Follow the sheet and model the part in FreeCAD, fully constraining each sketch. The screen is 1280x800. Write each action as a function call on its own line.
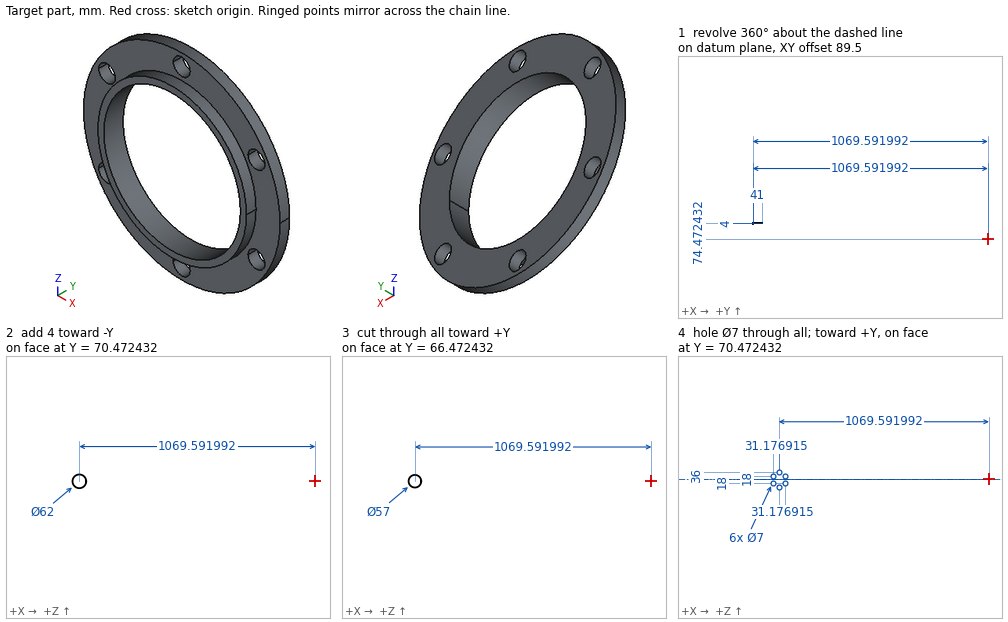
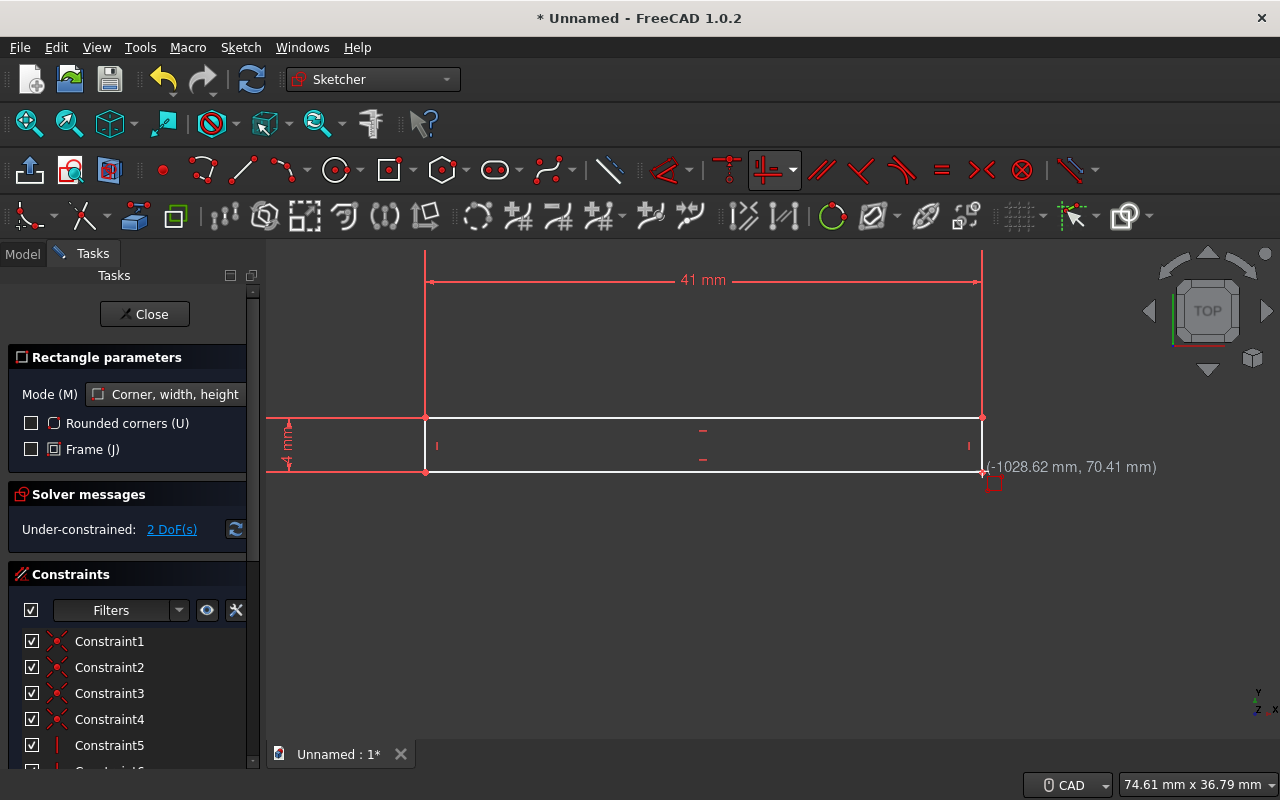
click(244, 170)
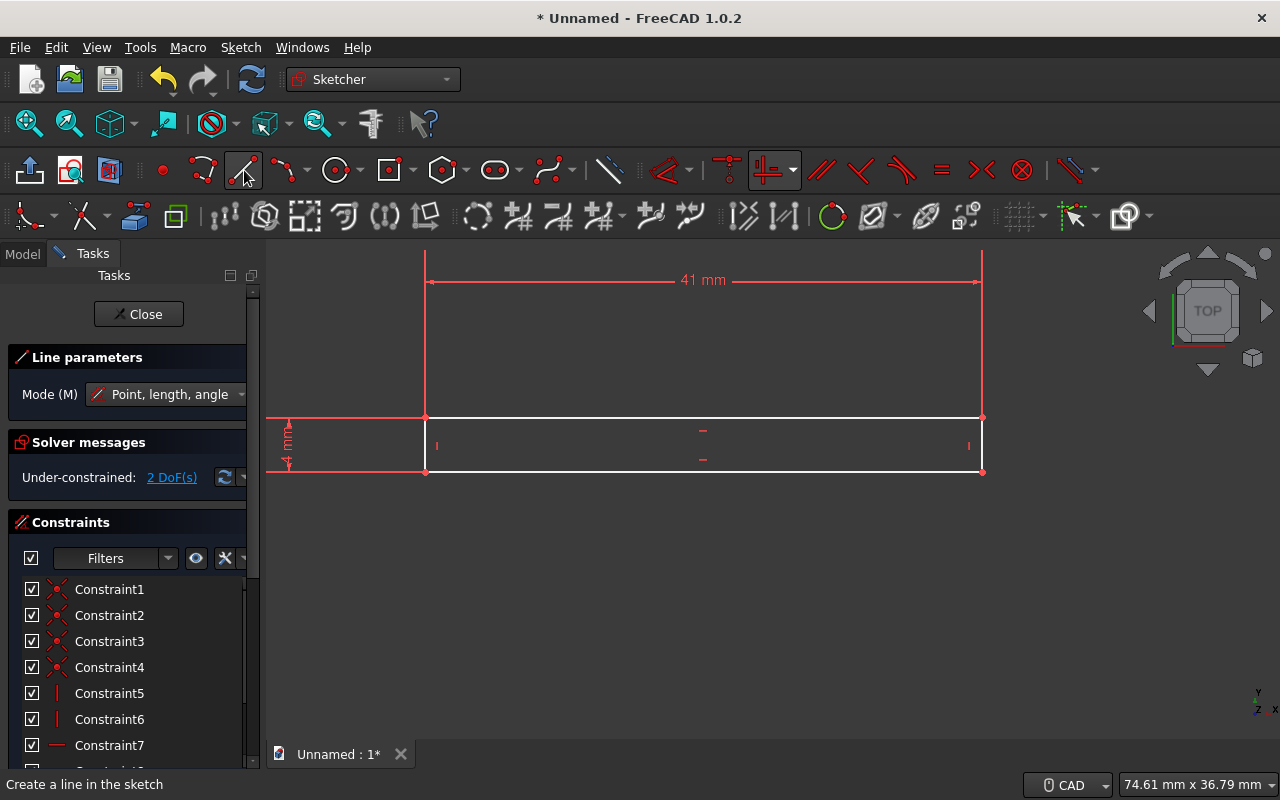
click(425, 493)
click(425, 560)
key(Escape)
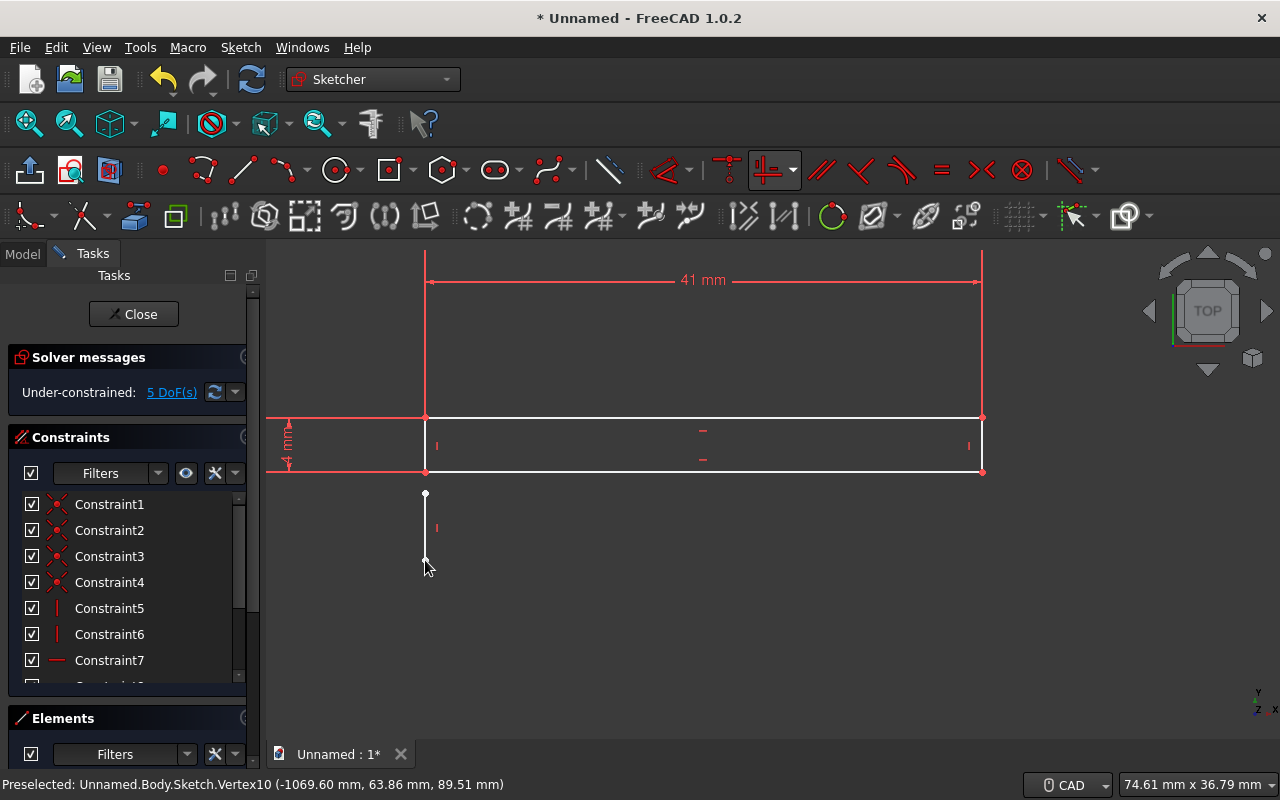
click(425, 514)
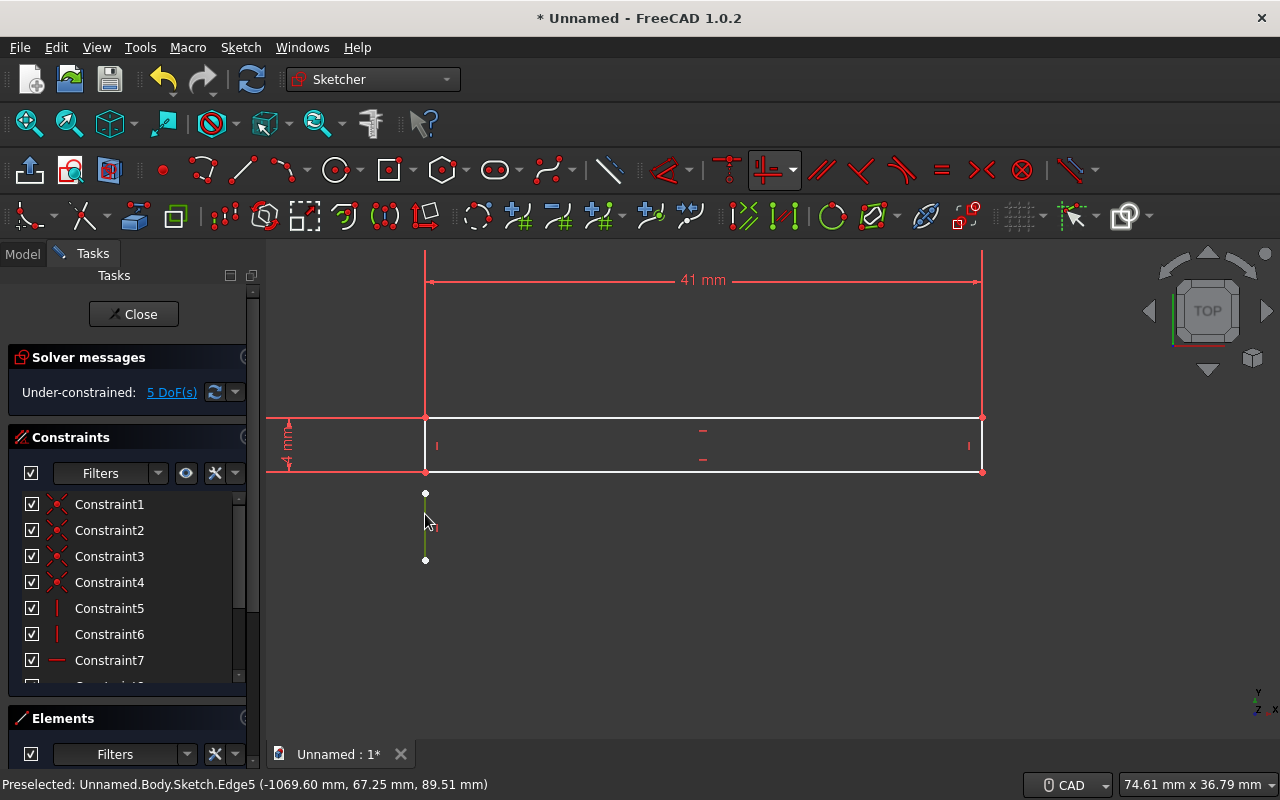
click(610, 170)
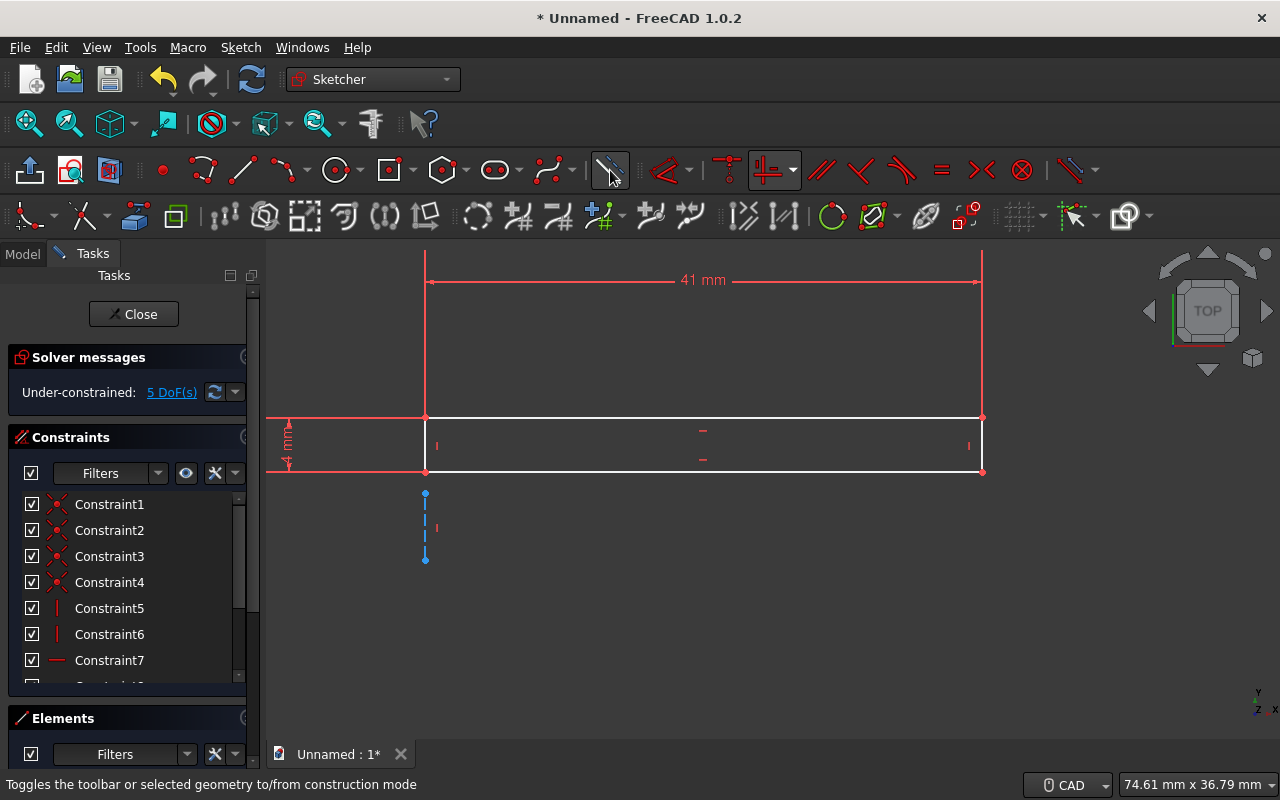
click(425, 418)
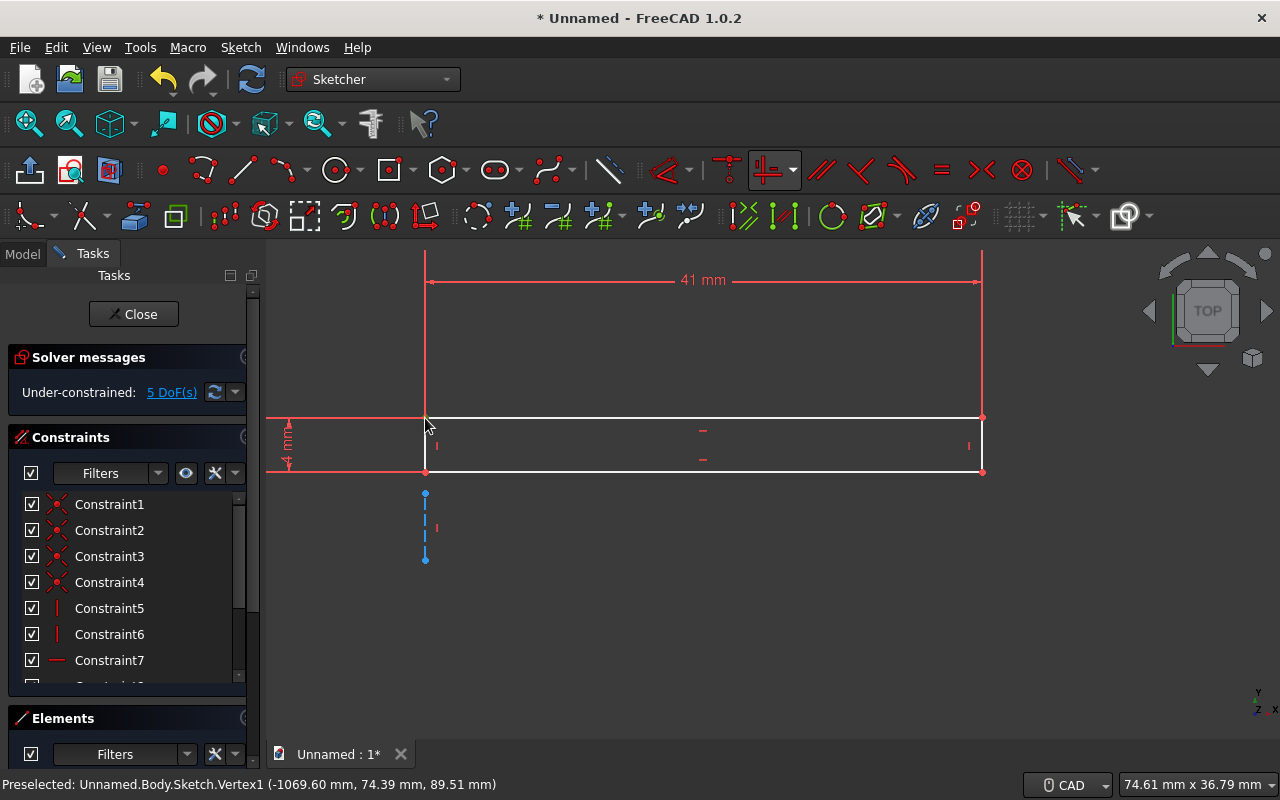
click(692, 170)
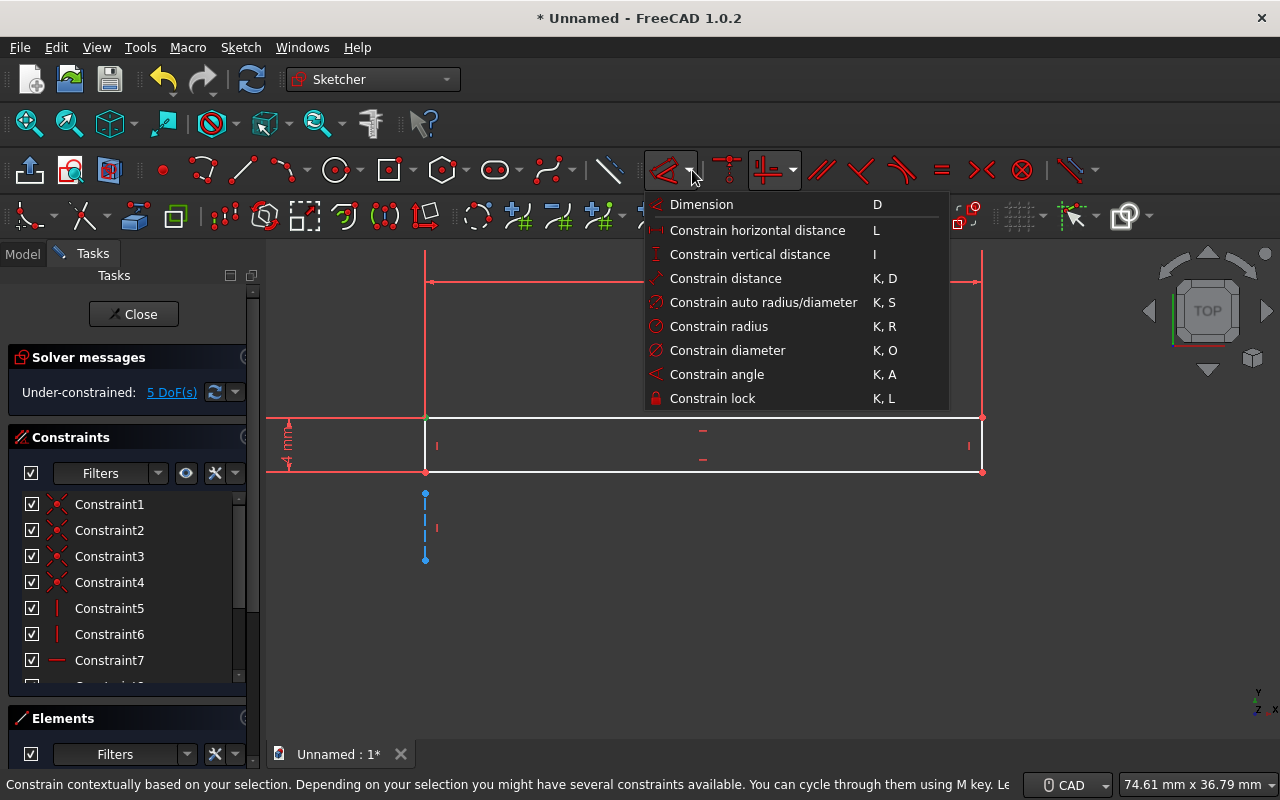
click(797, 254)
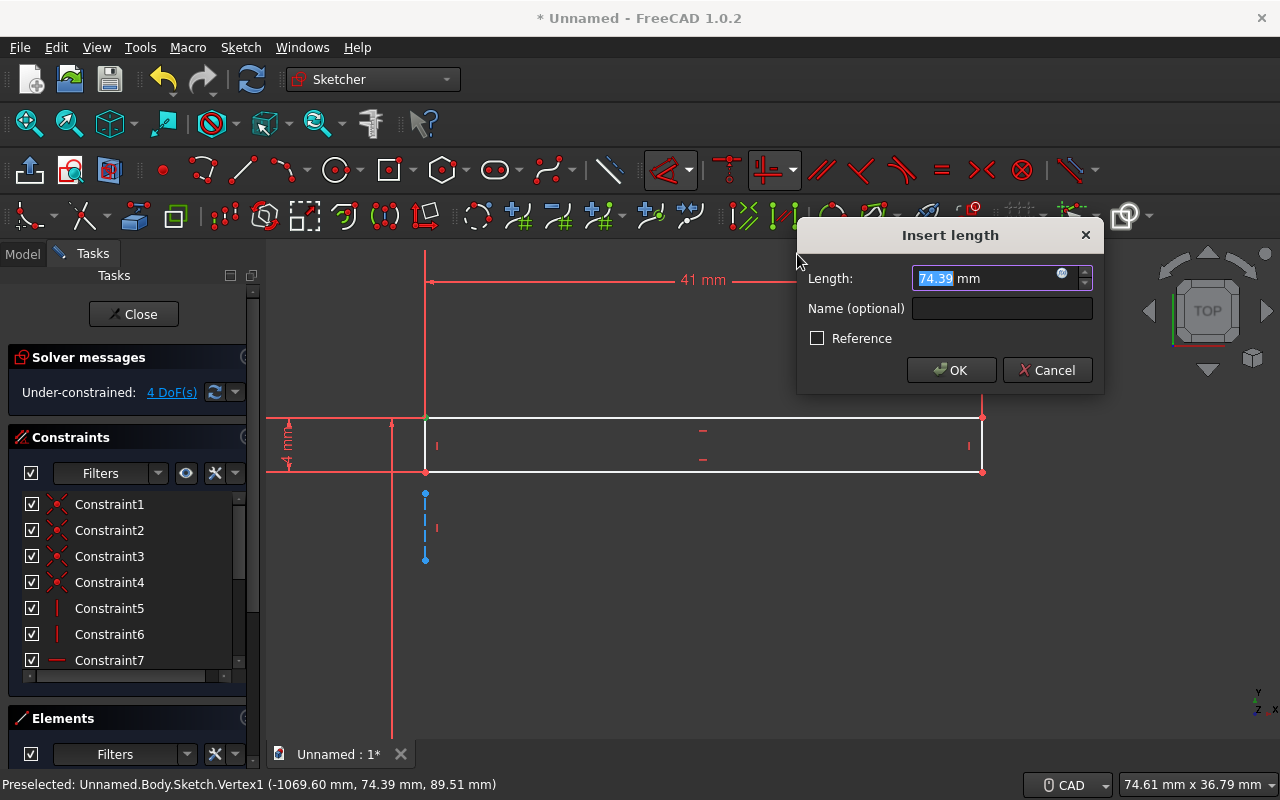
text(74.472432)
key(Return)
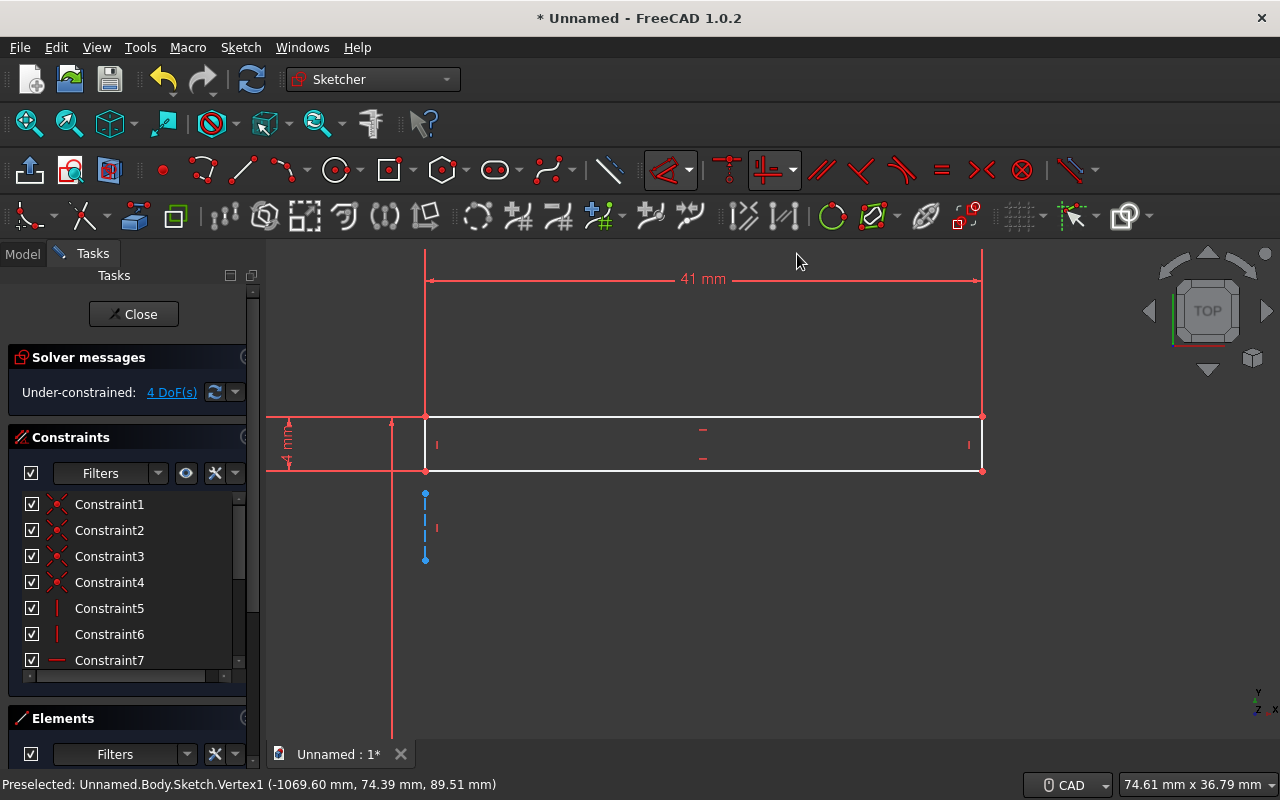
click(425, 417)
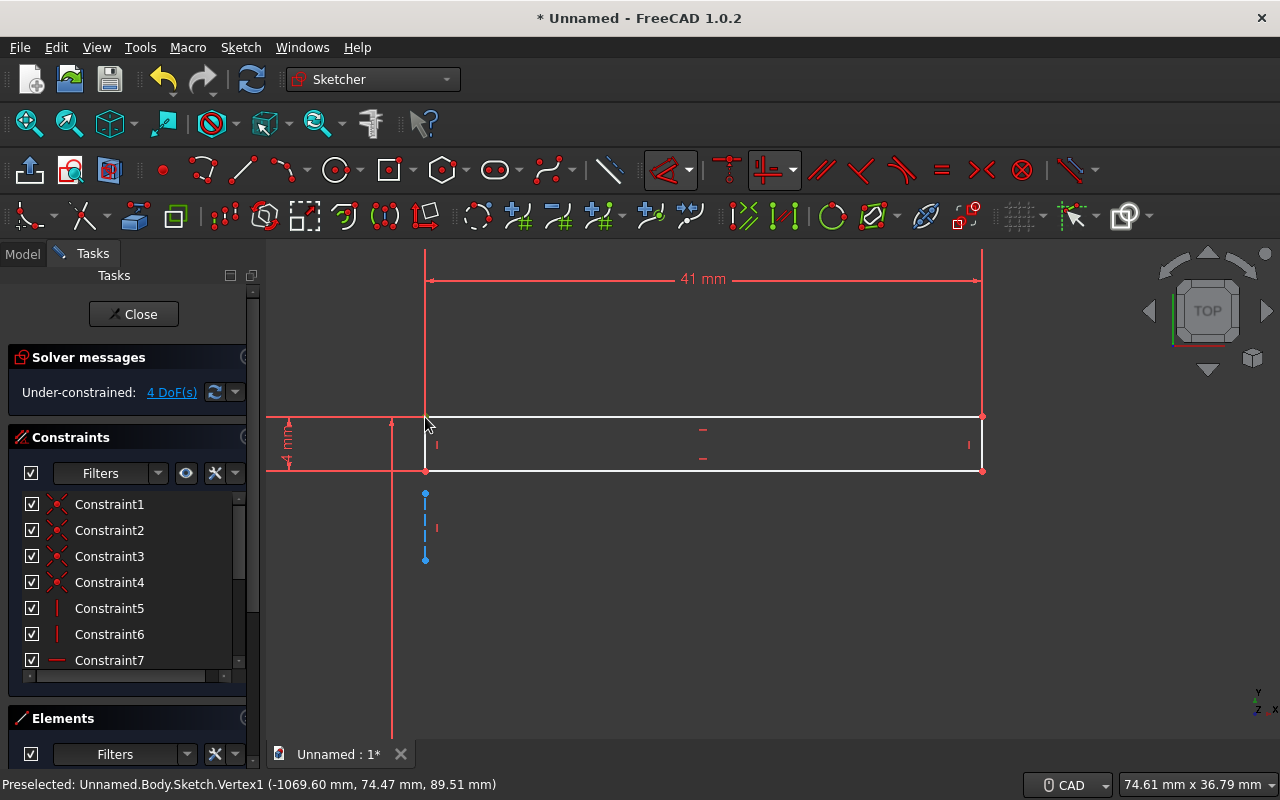
click(692, 170)